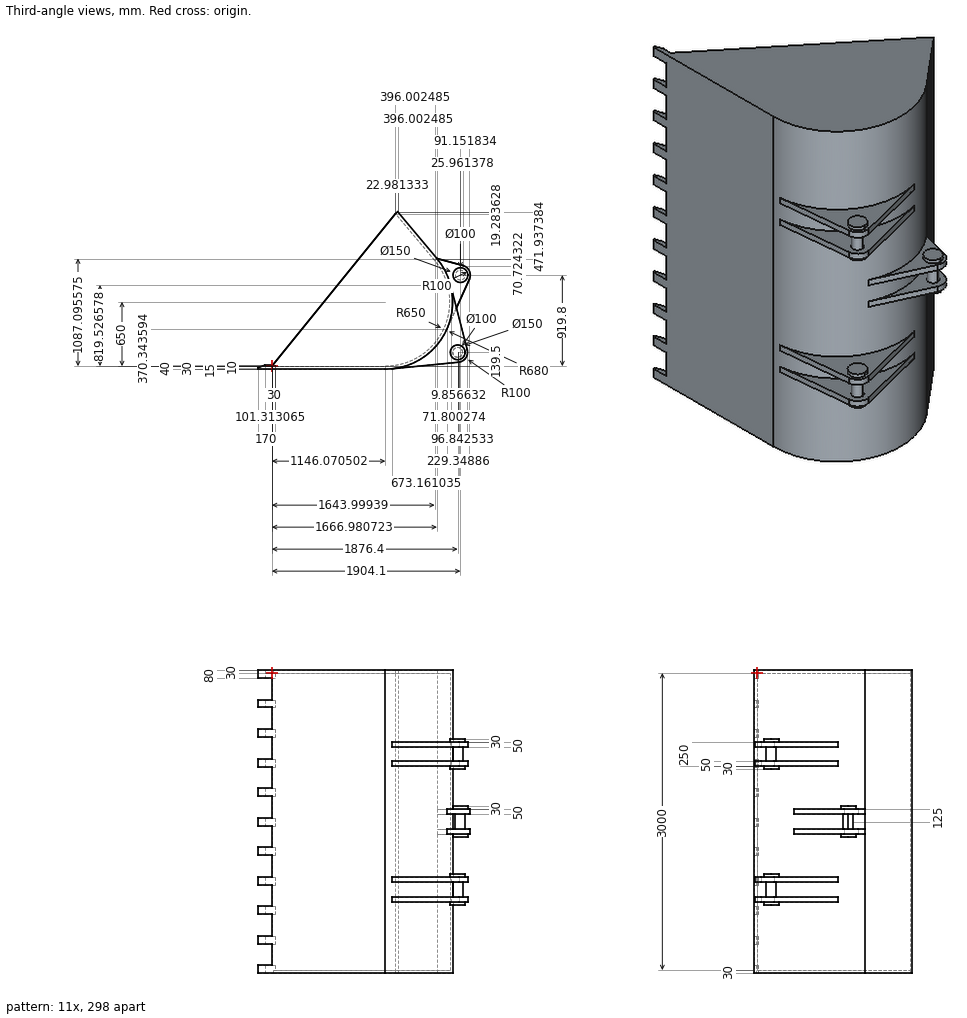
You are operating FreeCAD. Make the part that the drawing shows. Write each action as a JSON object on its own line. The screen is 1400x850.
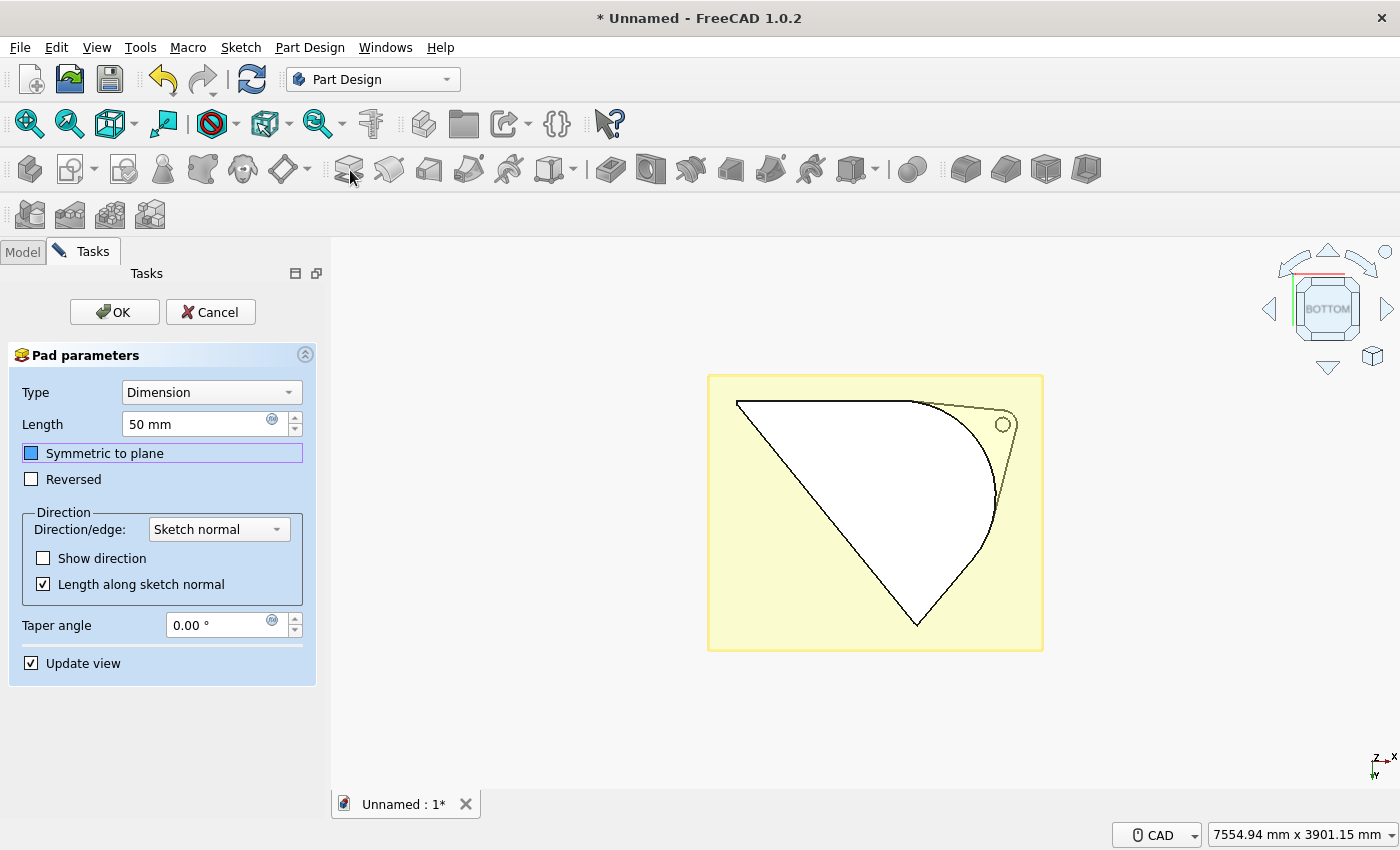
{"action": "left_click", "coordinate": [30, 479]}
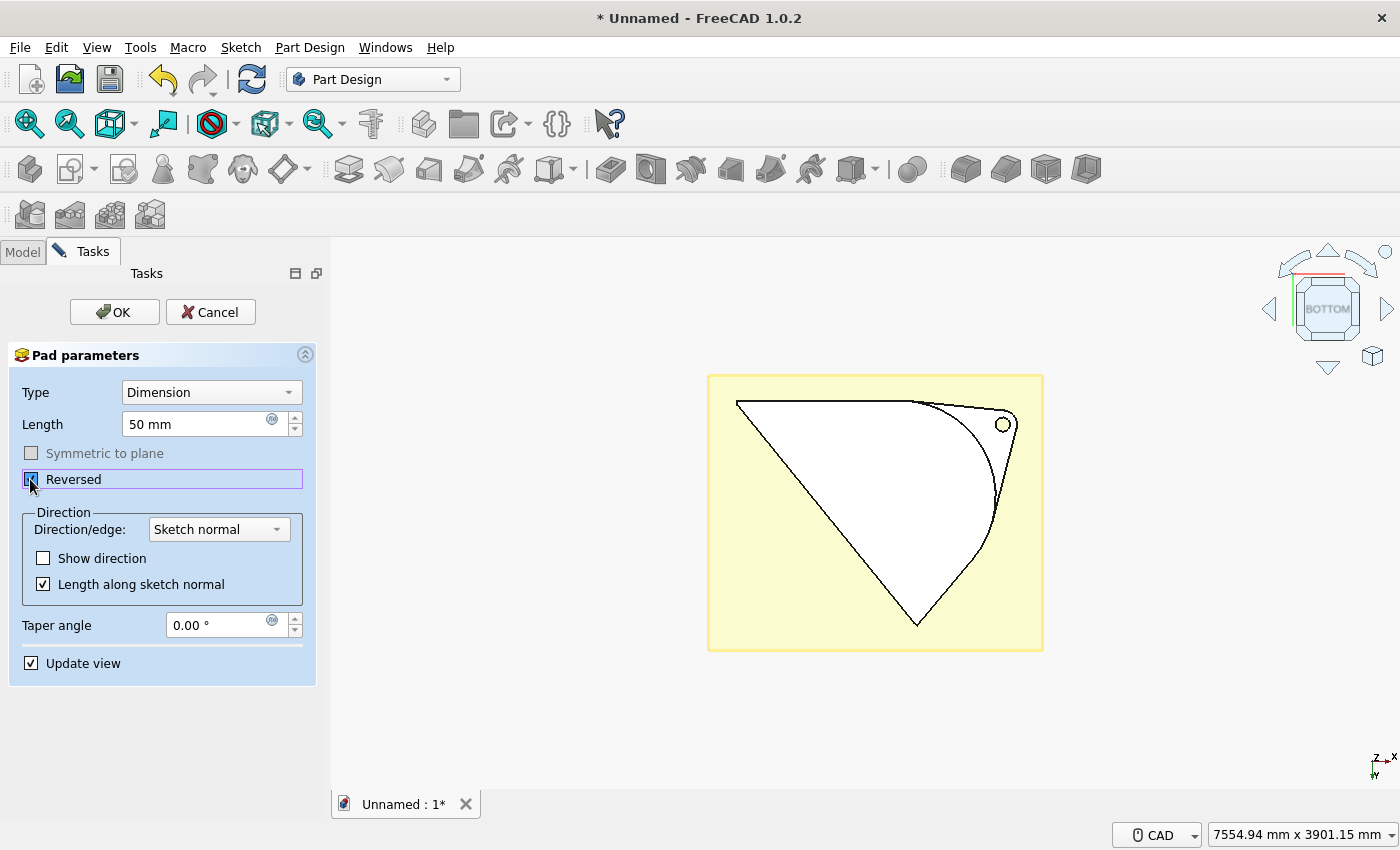
{"action": "left_click", "coordinate": [115, 312]}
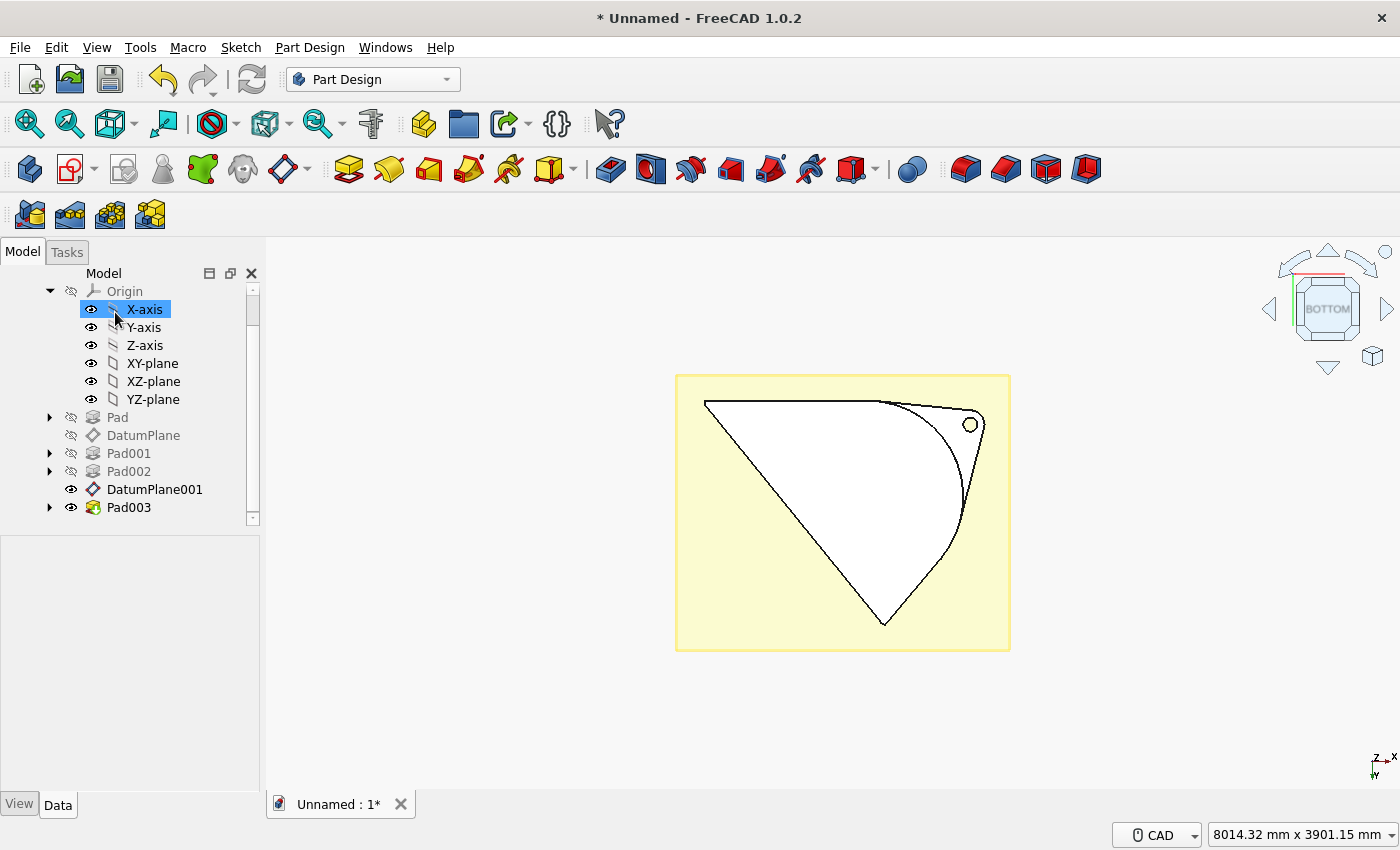
{"action": "left_click", "coordinate": [116, 489]}
{"action": "key", "text": "space"}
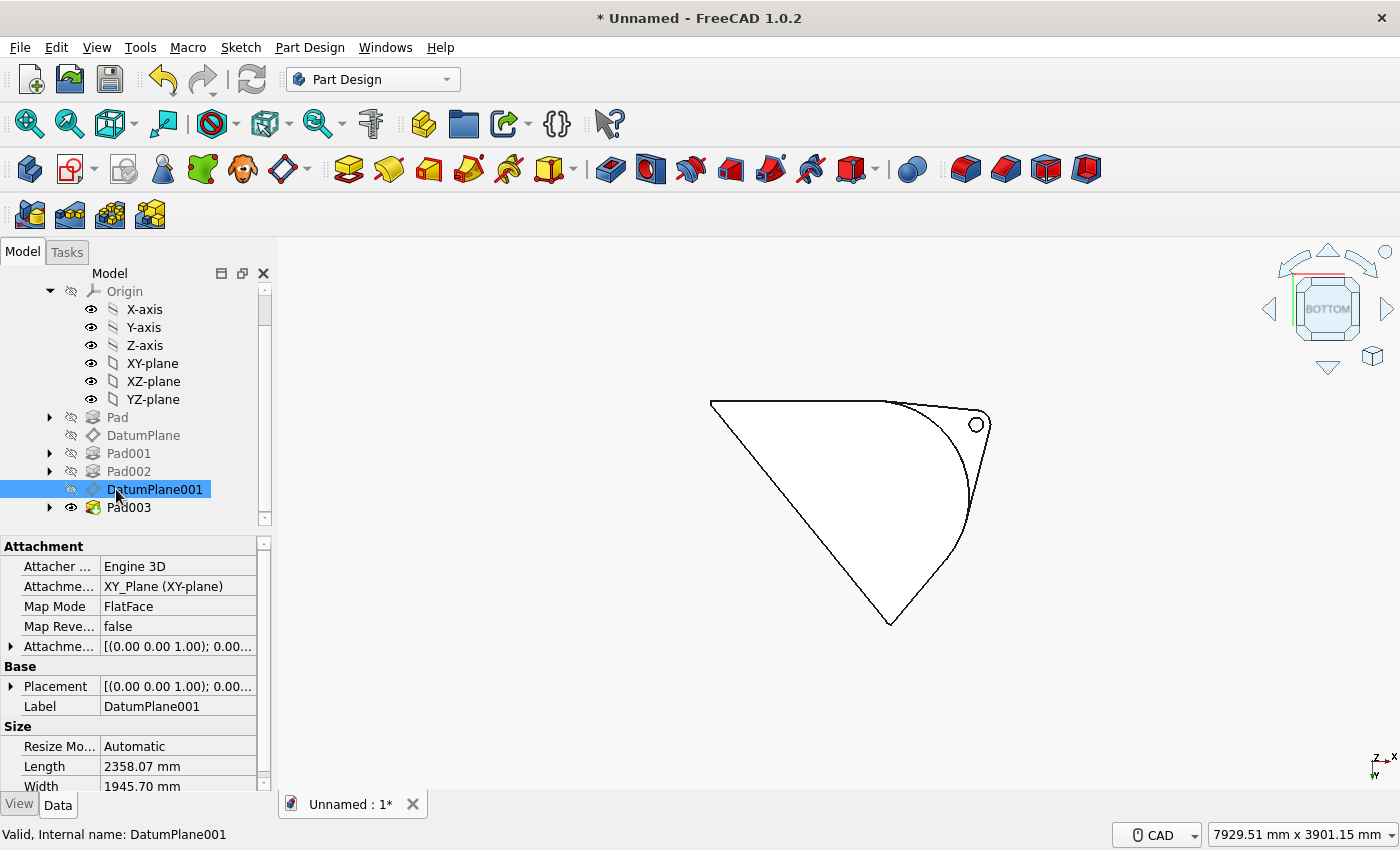
{"action": "left_click", "coordinate": [30, 124]}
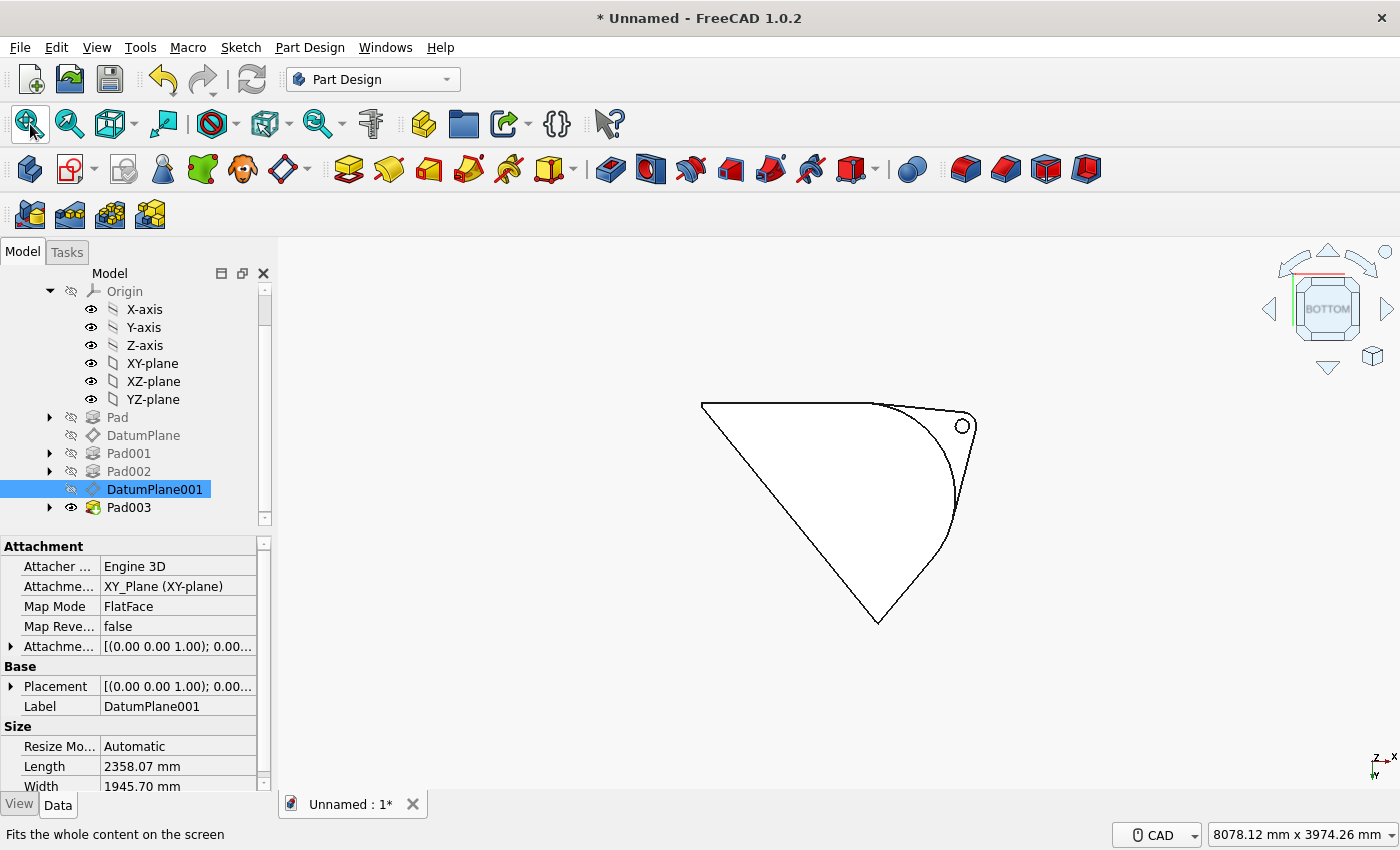
{"action": "left_click", "coordinate": [136, 363]}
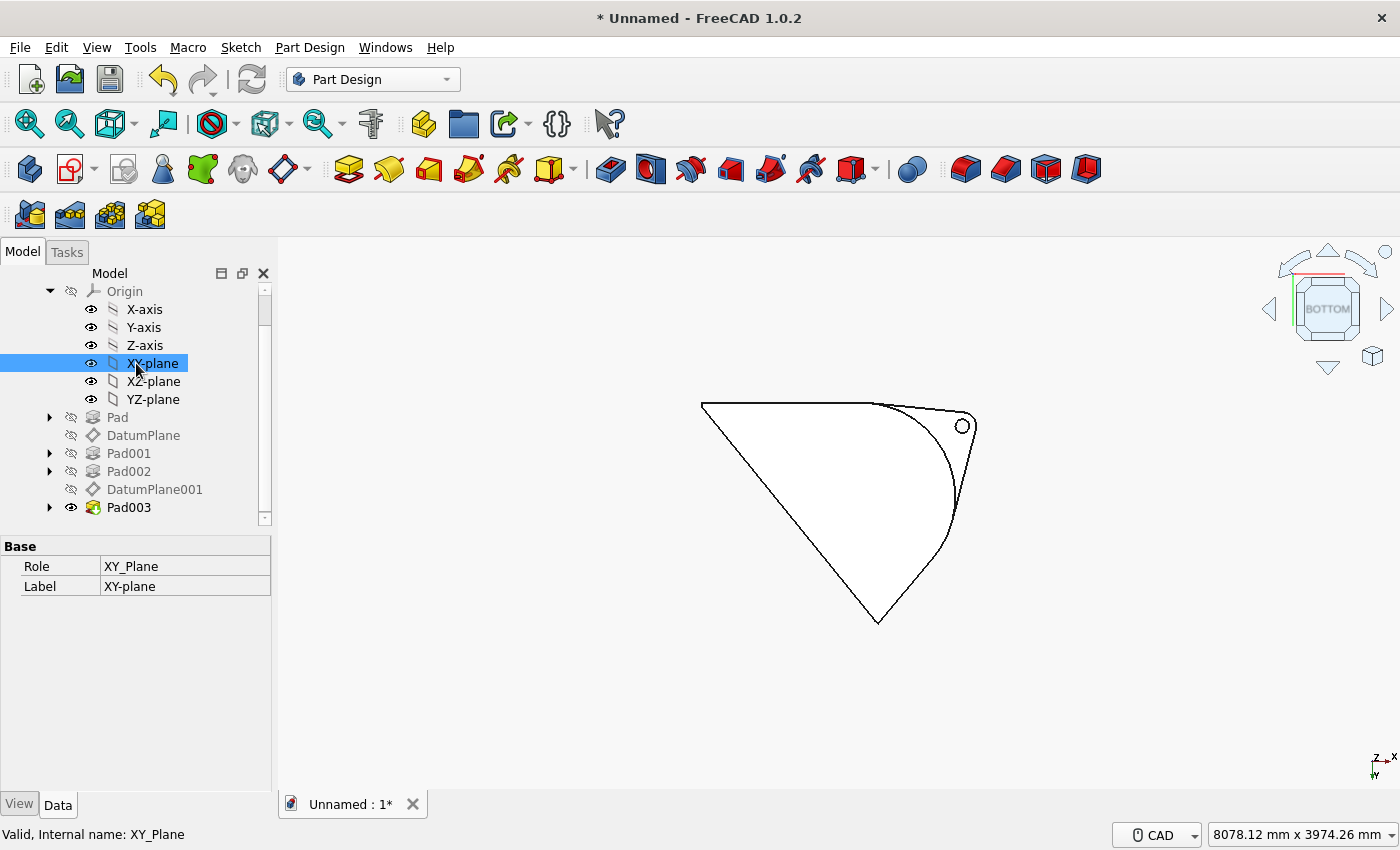
{"action": "left_click", "coordinate": [284, 170]}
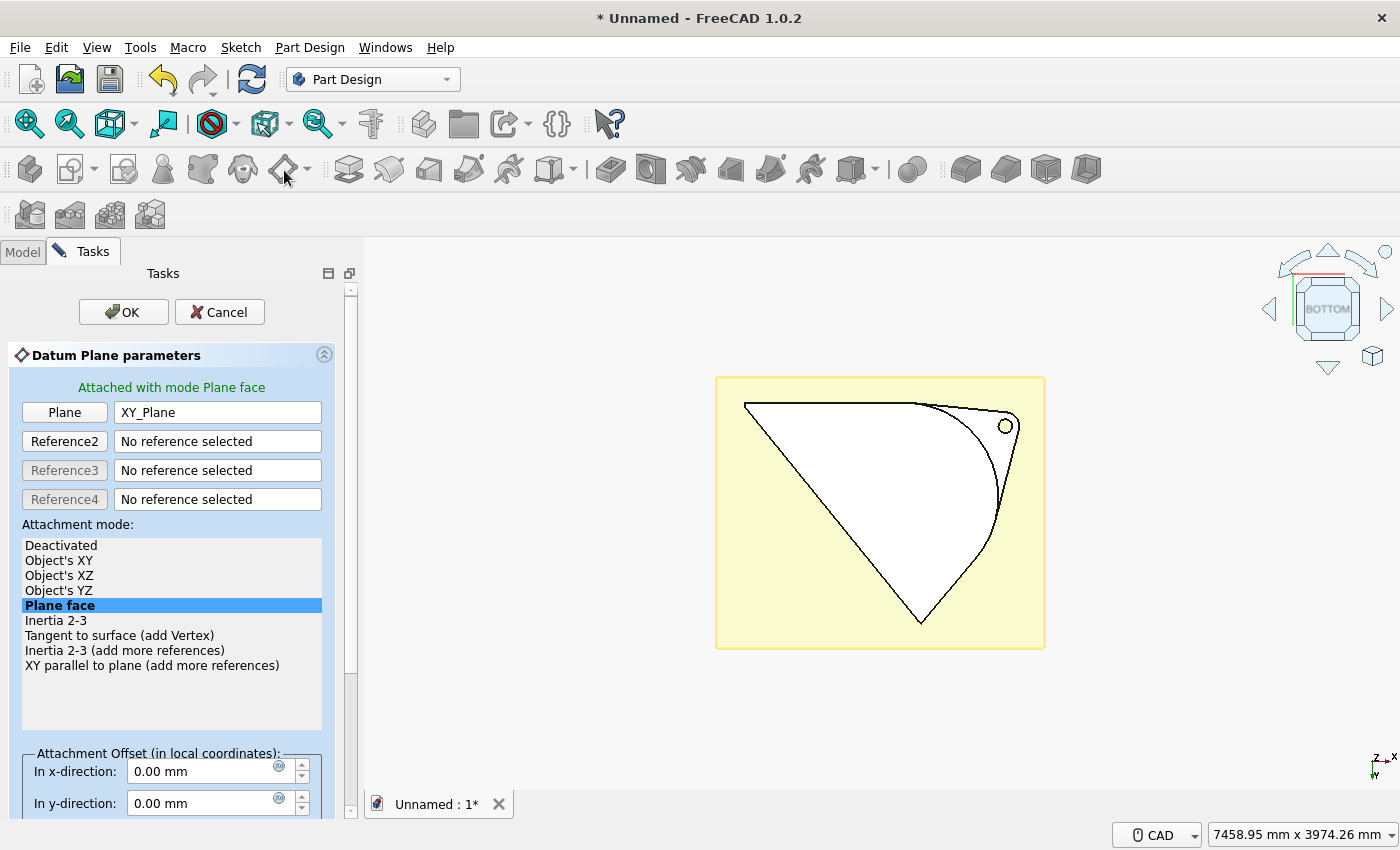
{"action": "scroll", "coordinate": [351, 550], "scroll_direction": "down", "scroll_amount": 2}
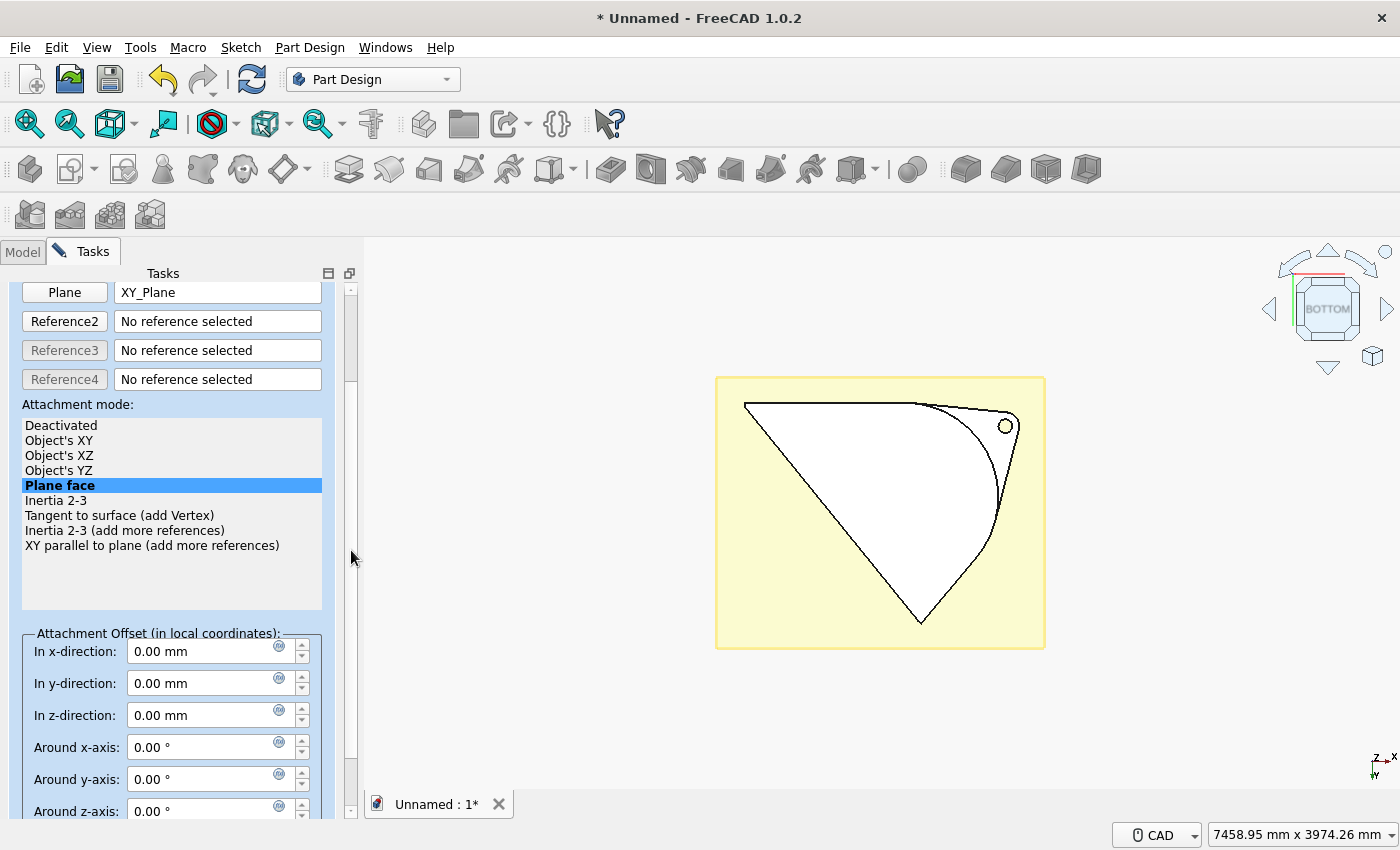
{"action": "triple_click", "coordinate": [210, 715]}